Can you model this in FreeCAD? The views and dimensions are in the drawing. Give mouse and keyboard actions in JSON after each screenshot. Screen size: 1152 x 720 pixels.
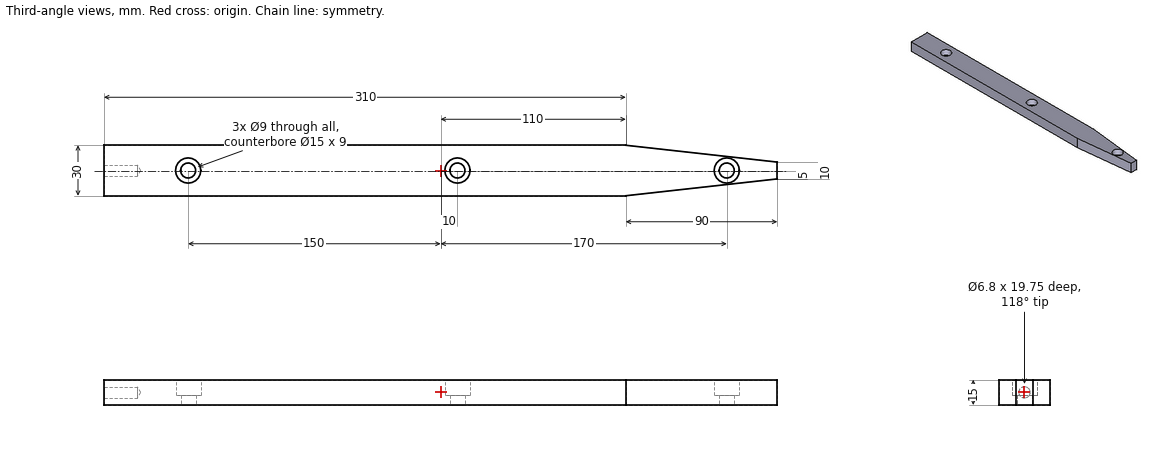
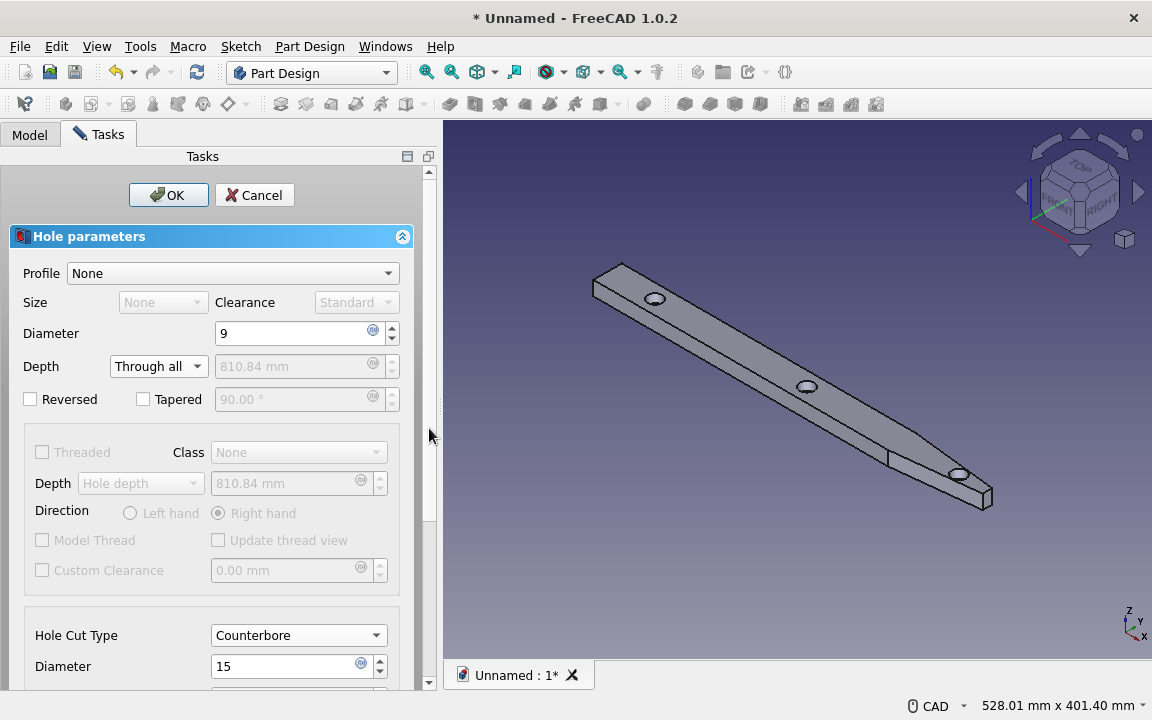
{"action": "left_click", "coordinate": [169, 195]}